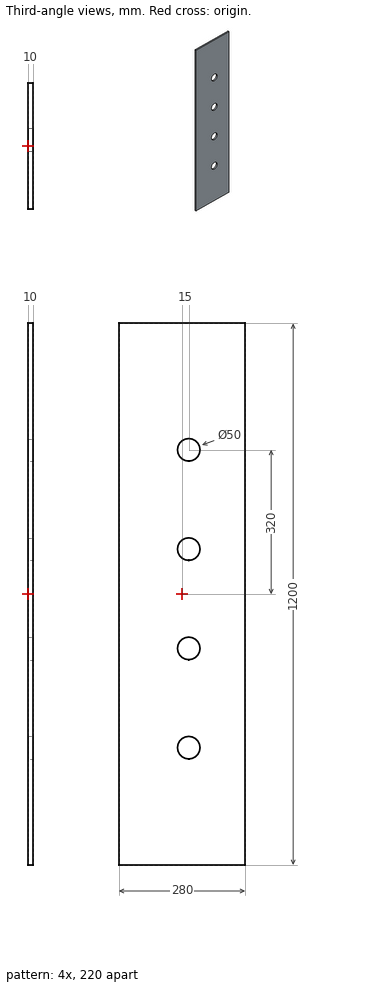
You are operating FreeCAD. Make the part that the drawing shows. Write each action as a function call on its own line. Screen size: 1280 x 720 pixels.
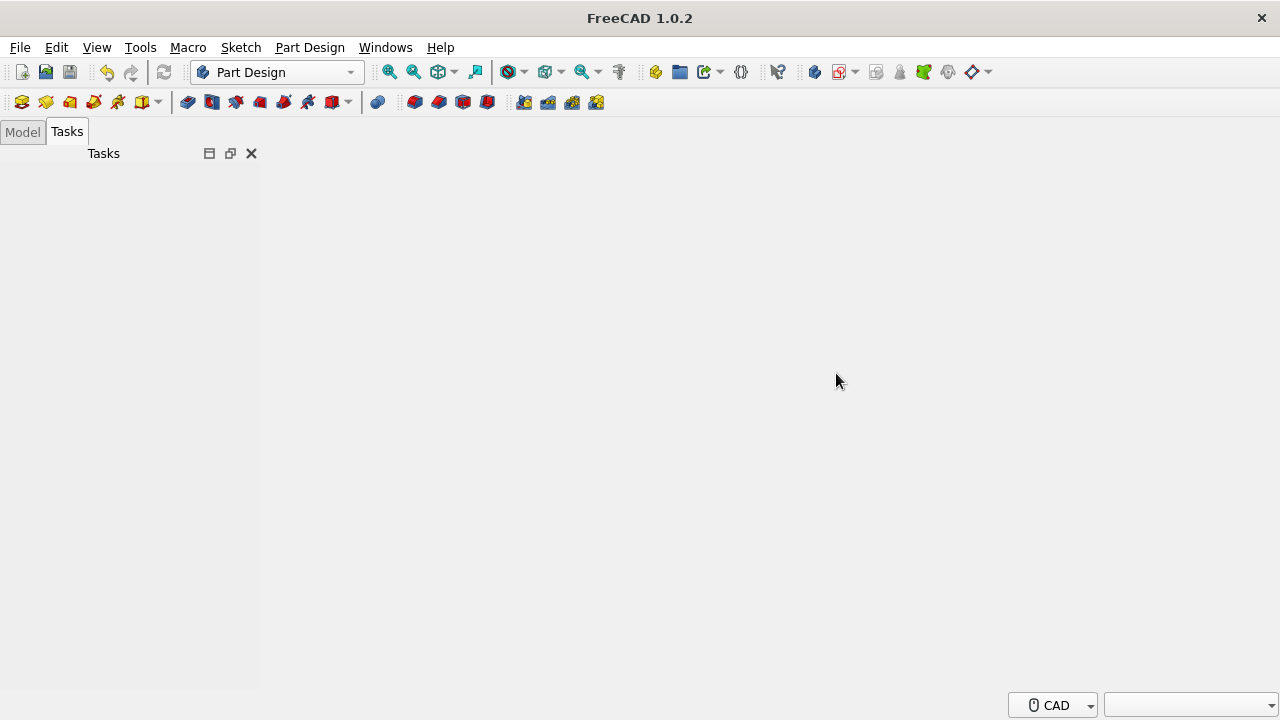
click(22, 72)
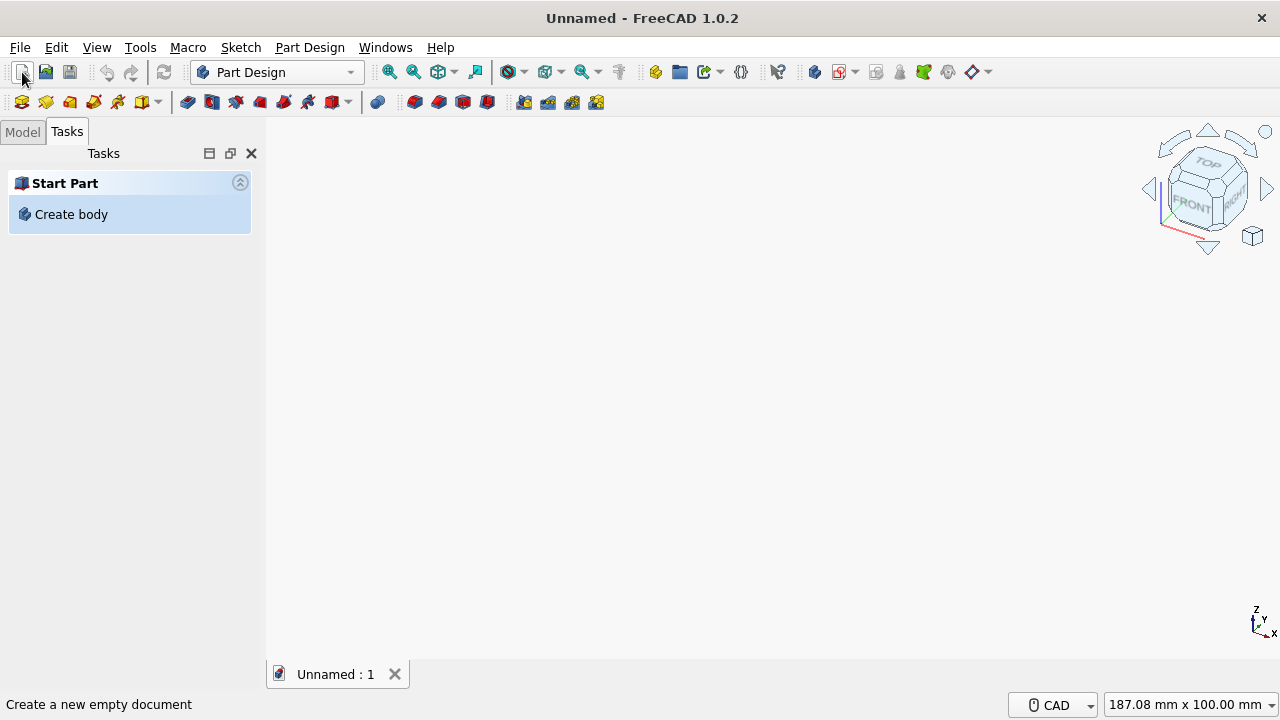
click(840, 72)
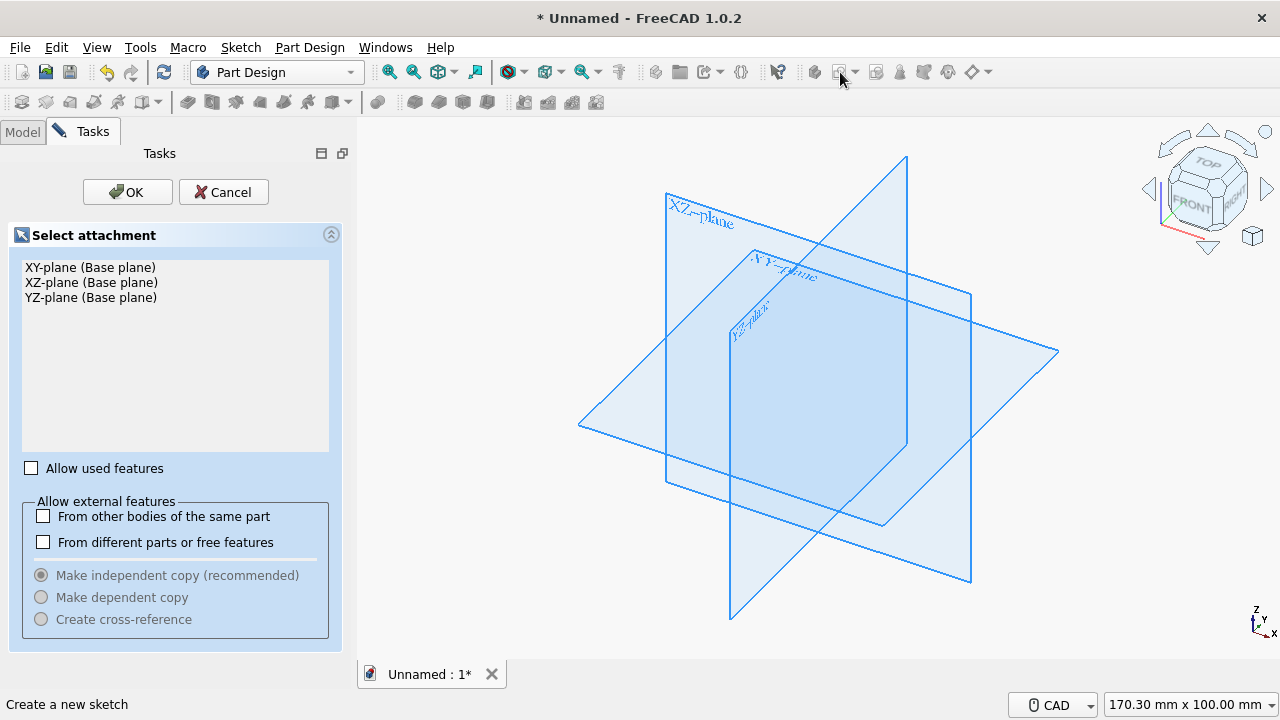
click(82, 298)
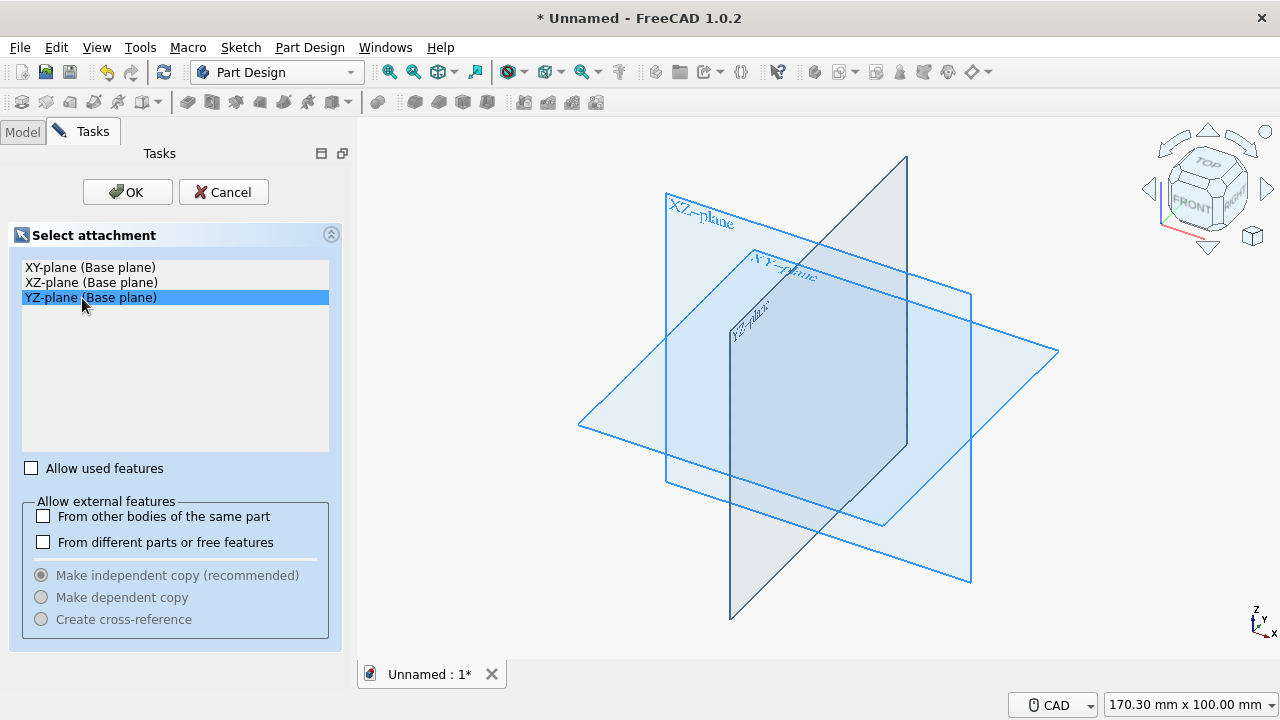
click(128, 192)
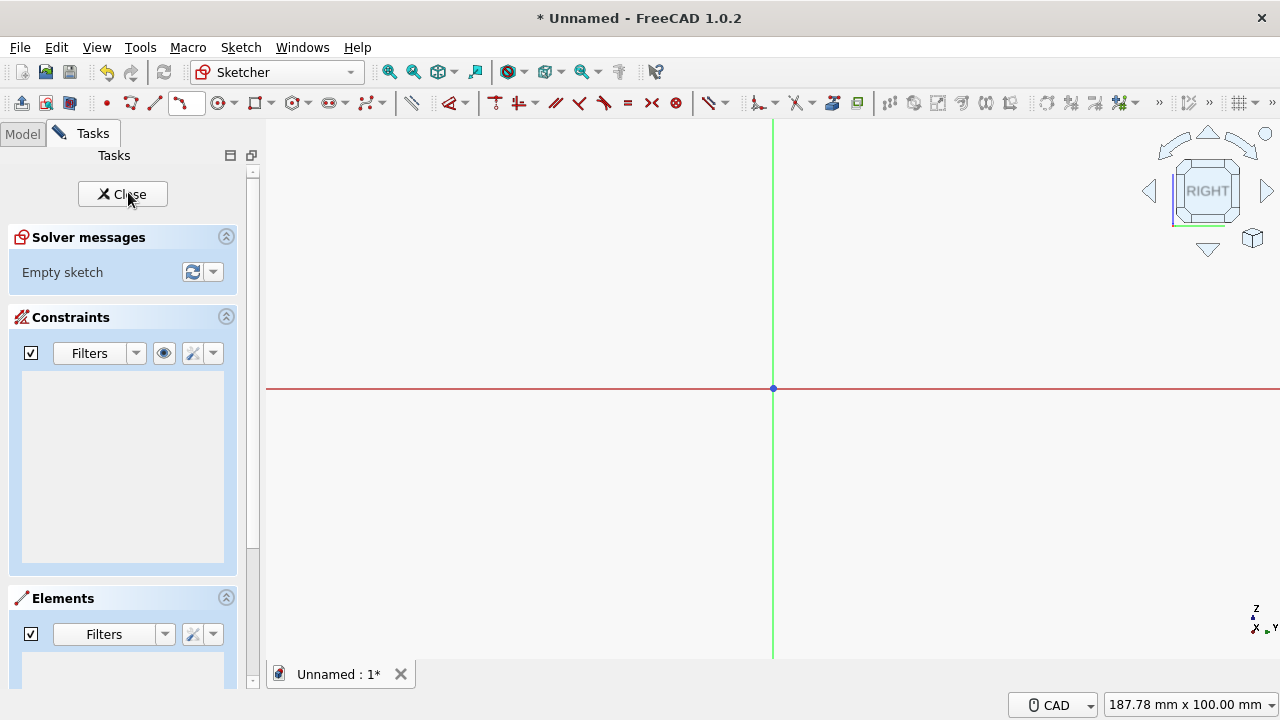
scroll(701, 389, down, 15)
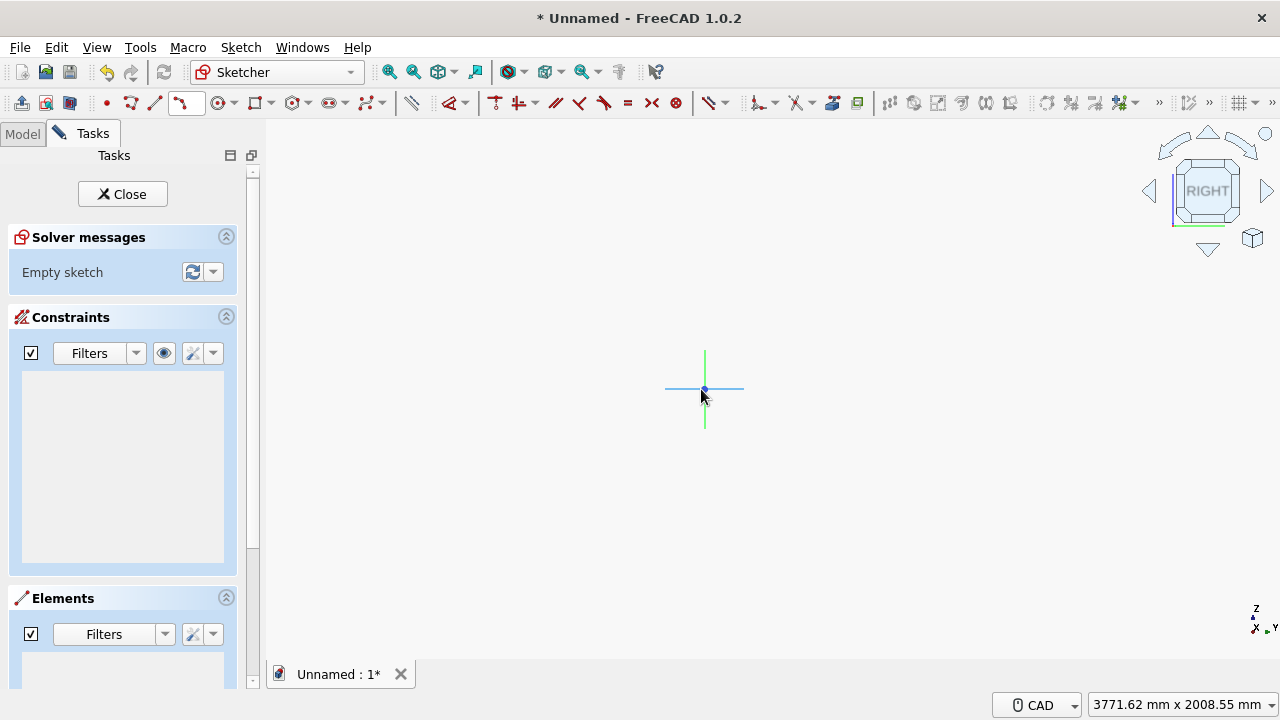
click(274, 104)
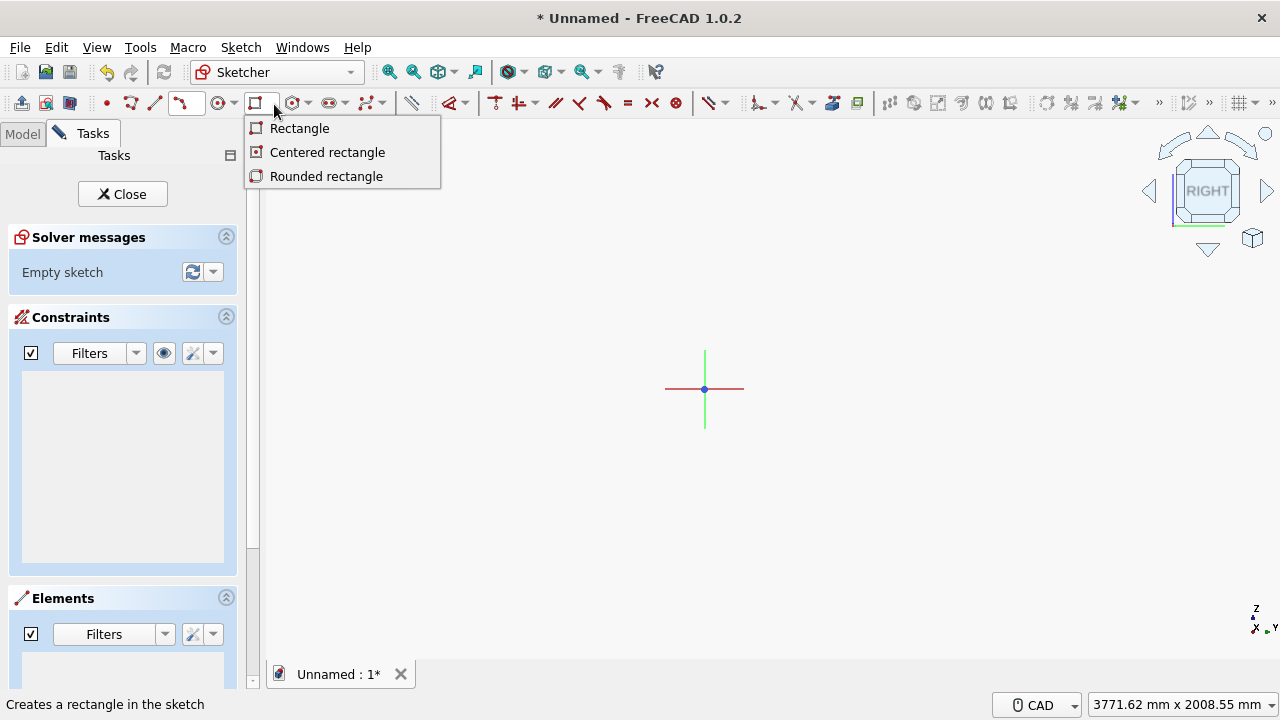
click(342, 152)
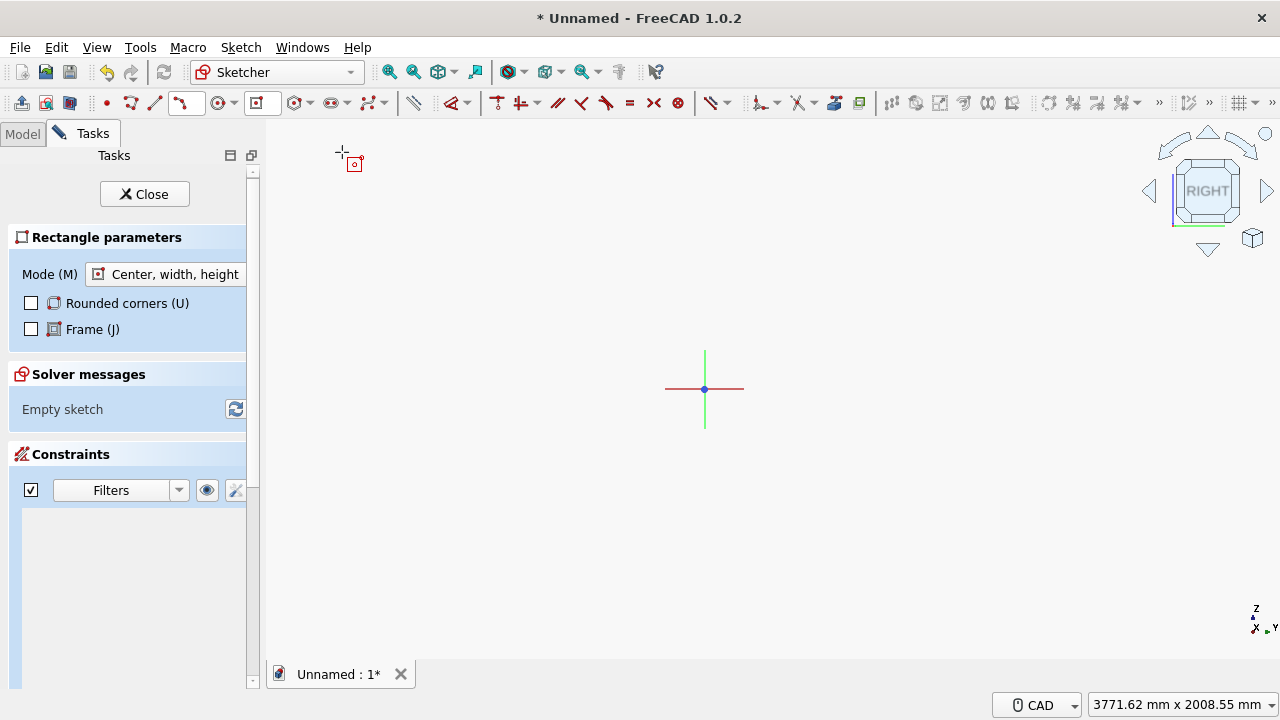
click(705, 389)
click(743, 228)
key(Escape)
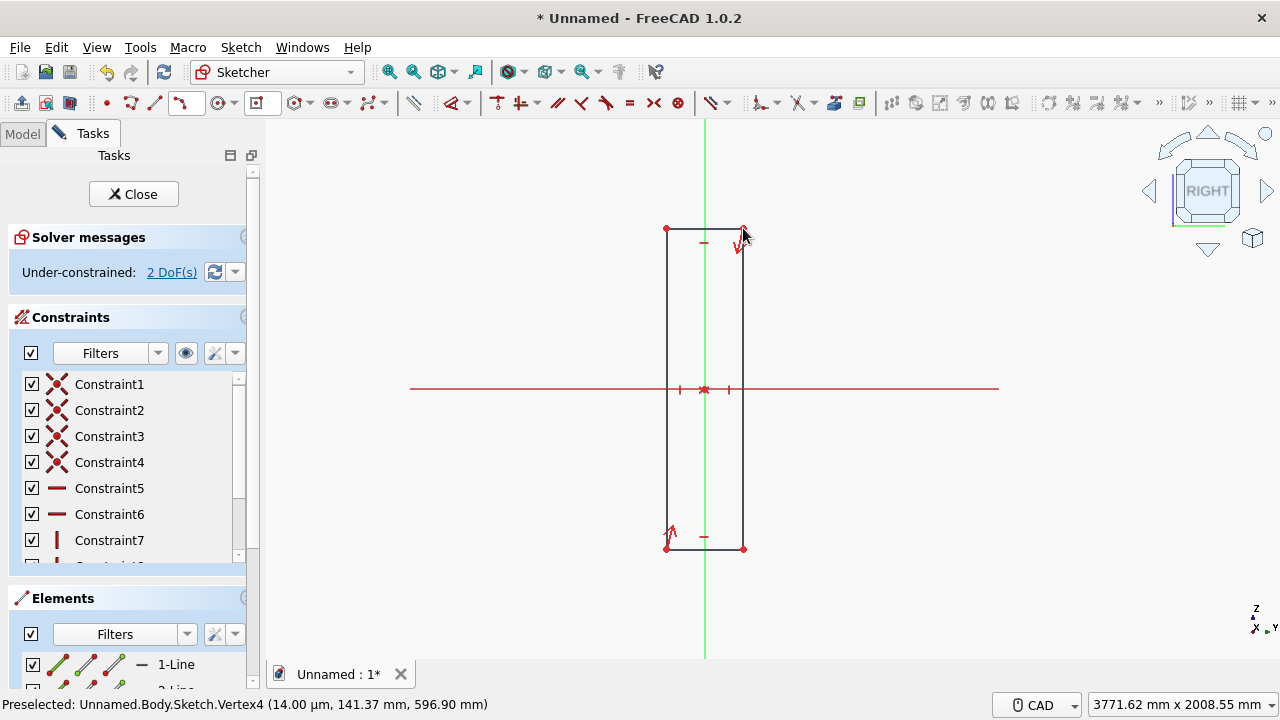
click(452, 104)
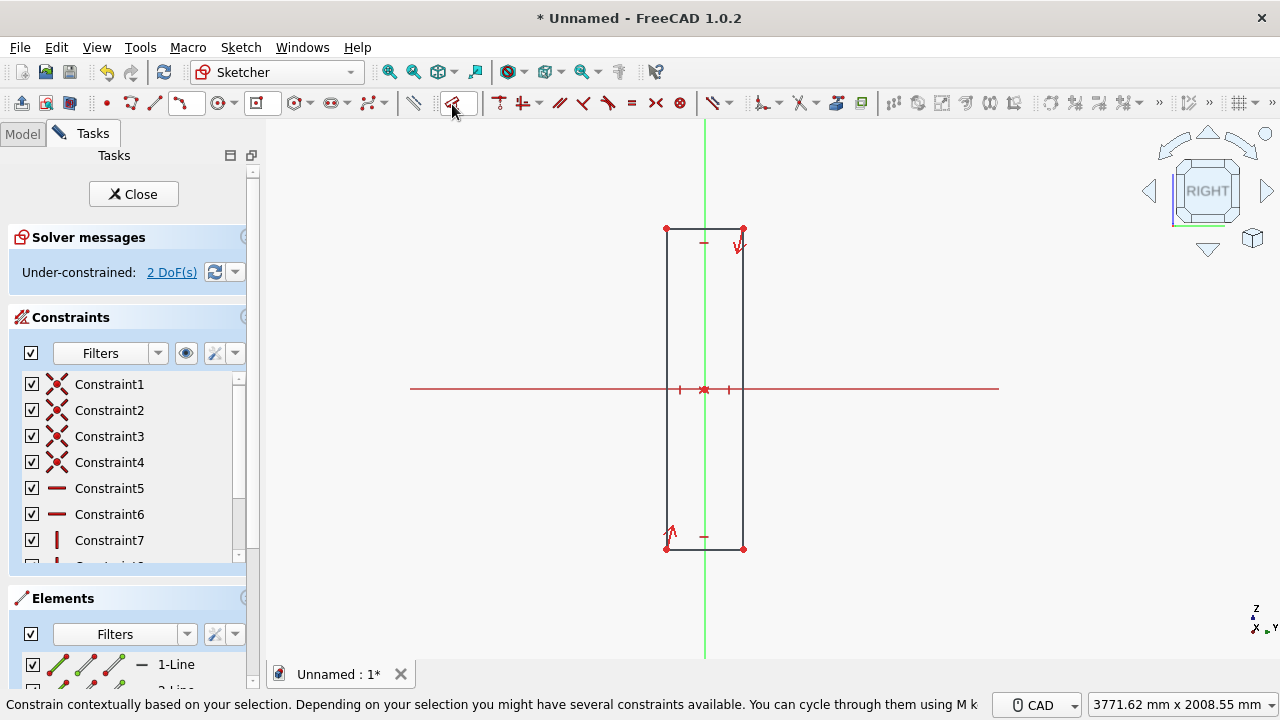
click(690, 550)
click(688, 584)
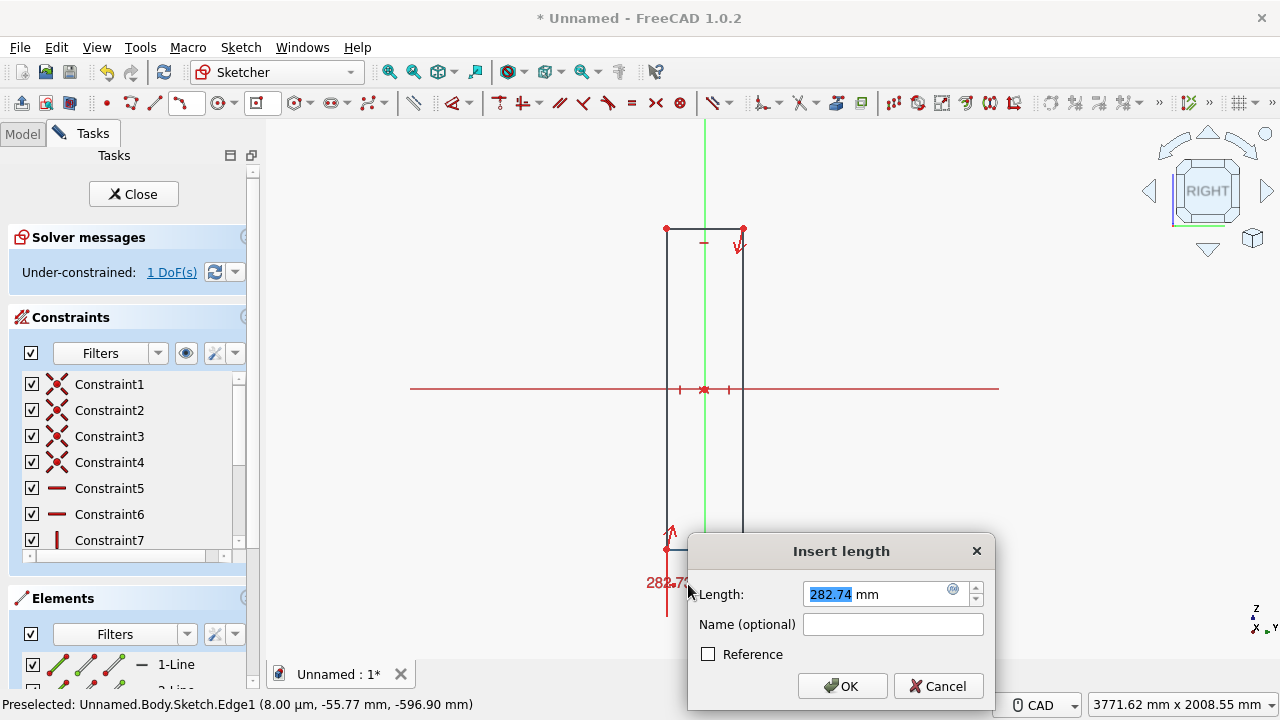
text(280)
key(Return)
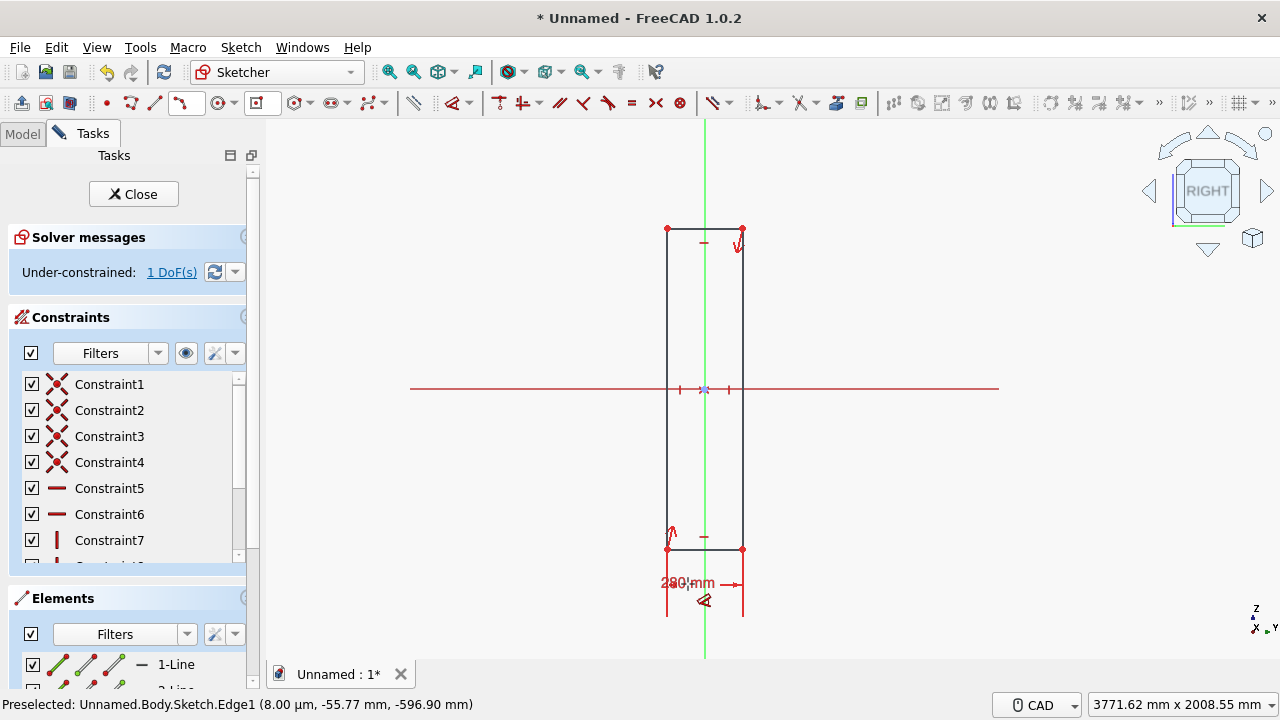
click(743, 454)
click(777, 316)